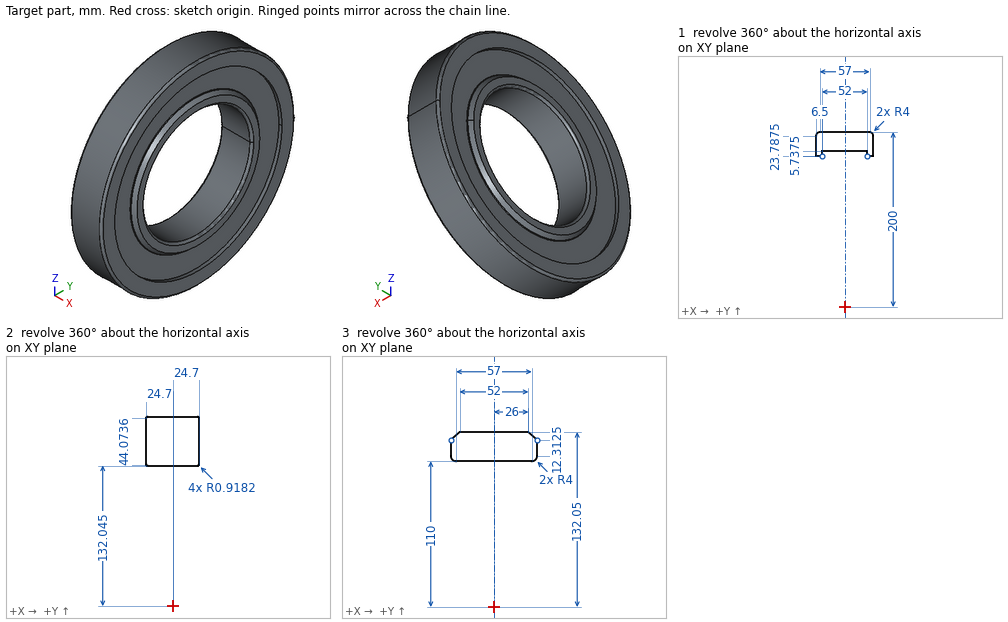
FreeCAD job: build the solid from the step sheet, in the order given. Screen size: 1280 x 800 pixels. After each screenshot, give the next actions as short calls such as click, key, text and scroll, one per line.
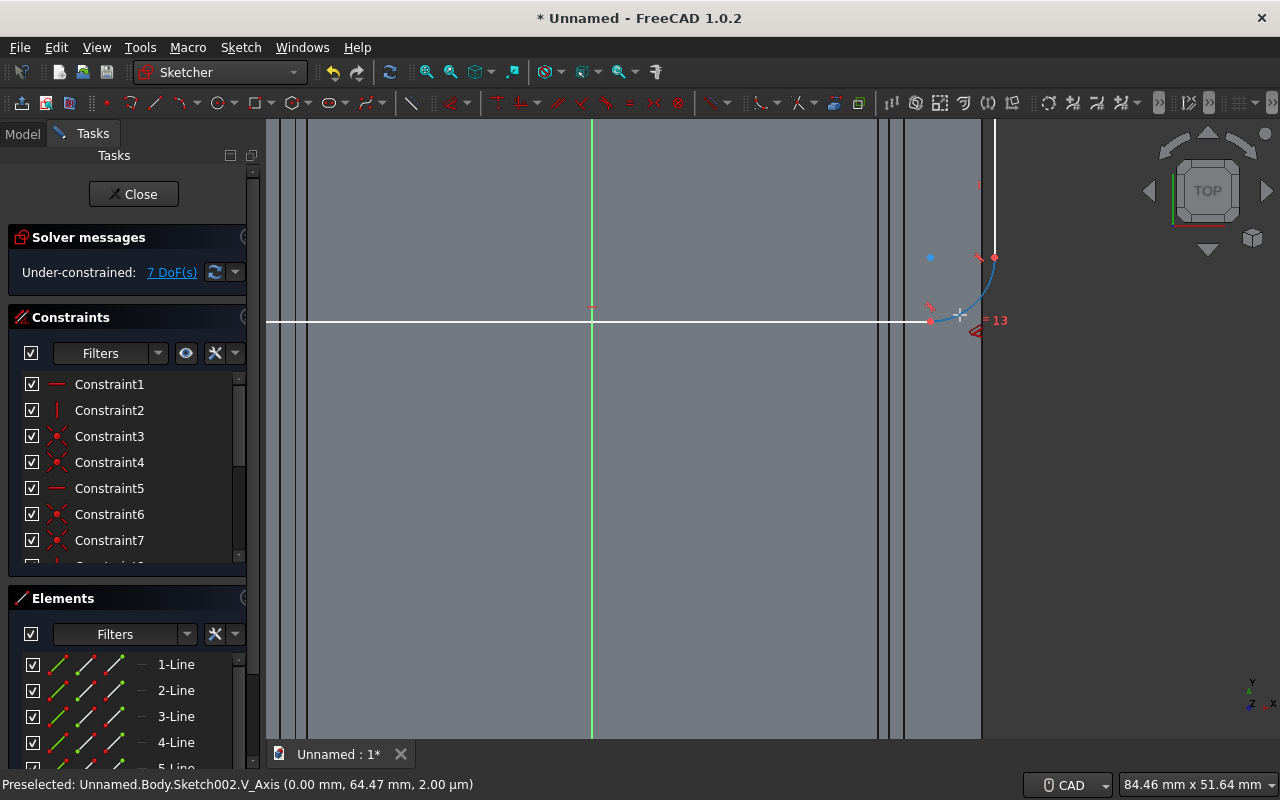
click(960, 315)
click(975, 343)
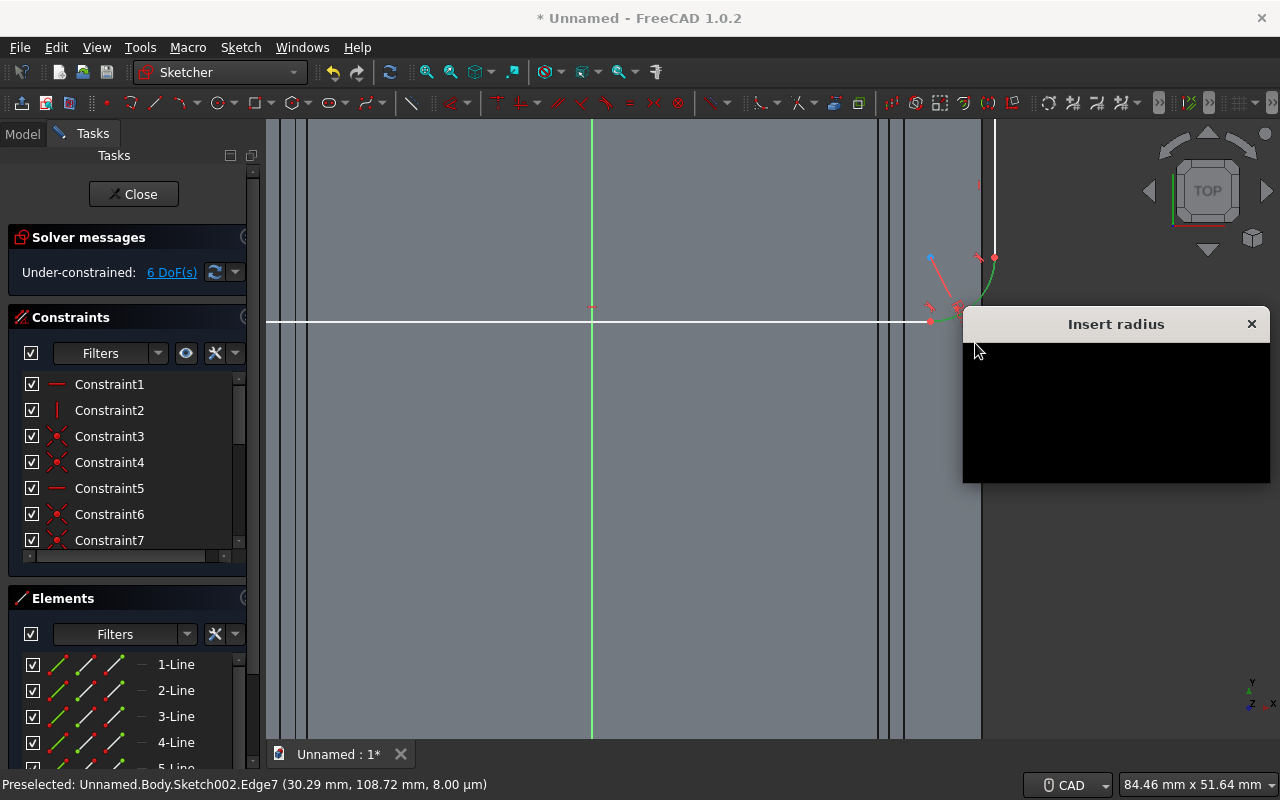
text(4)
key(Return)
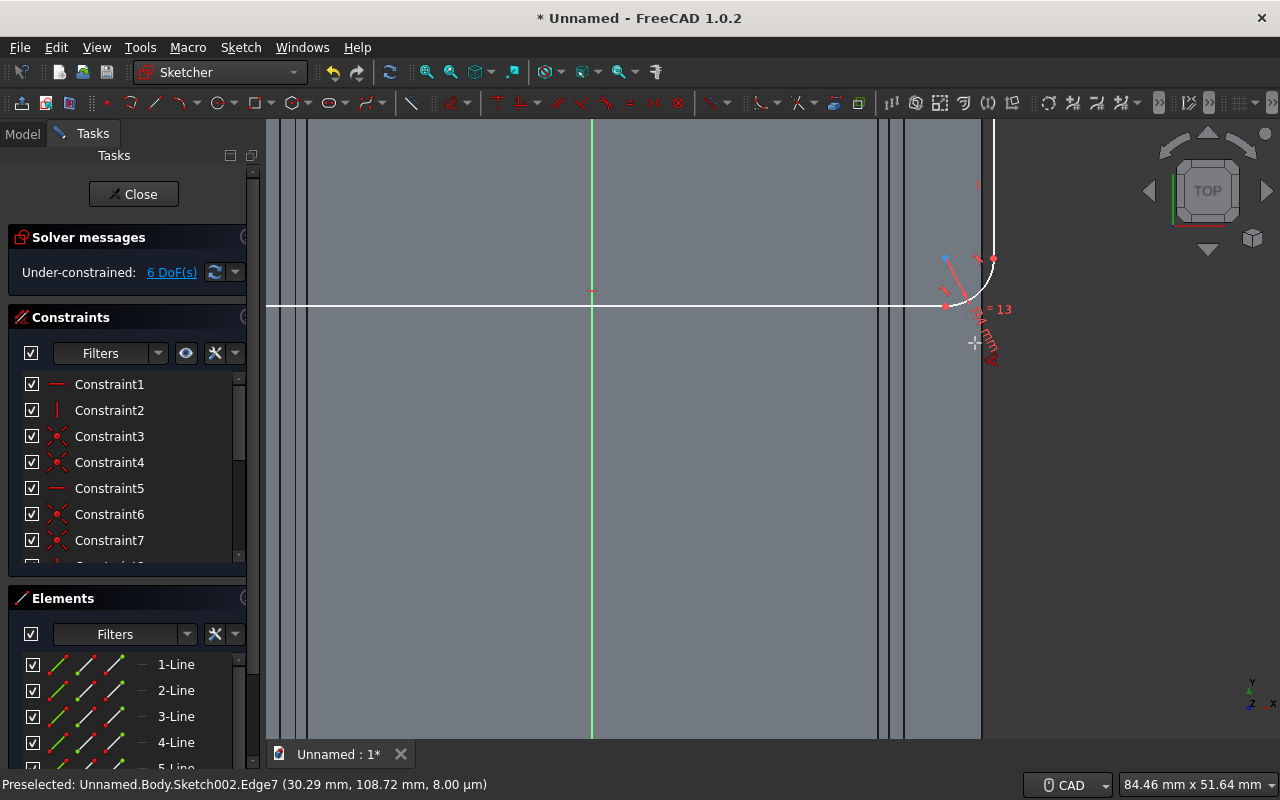
scroll(741, 298, down, 7)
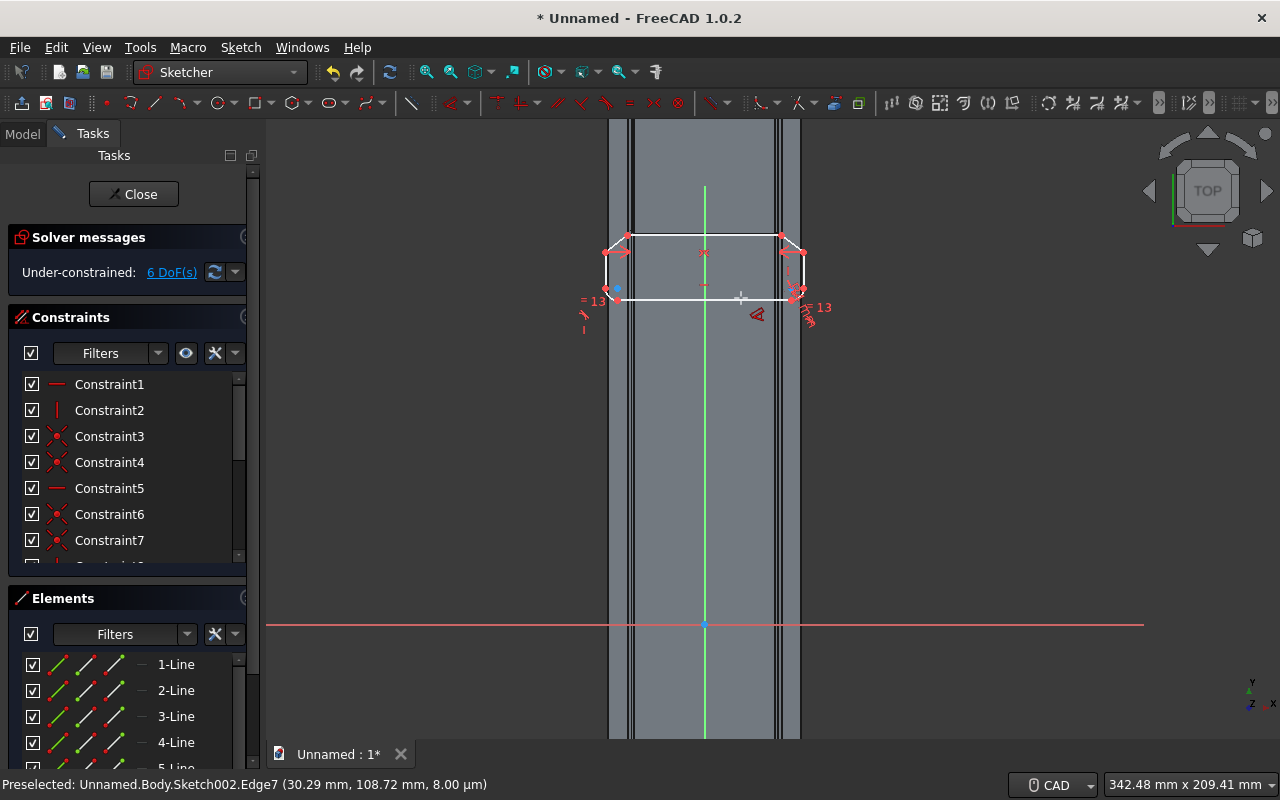
click(670, 300)
click(665, 266)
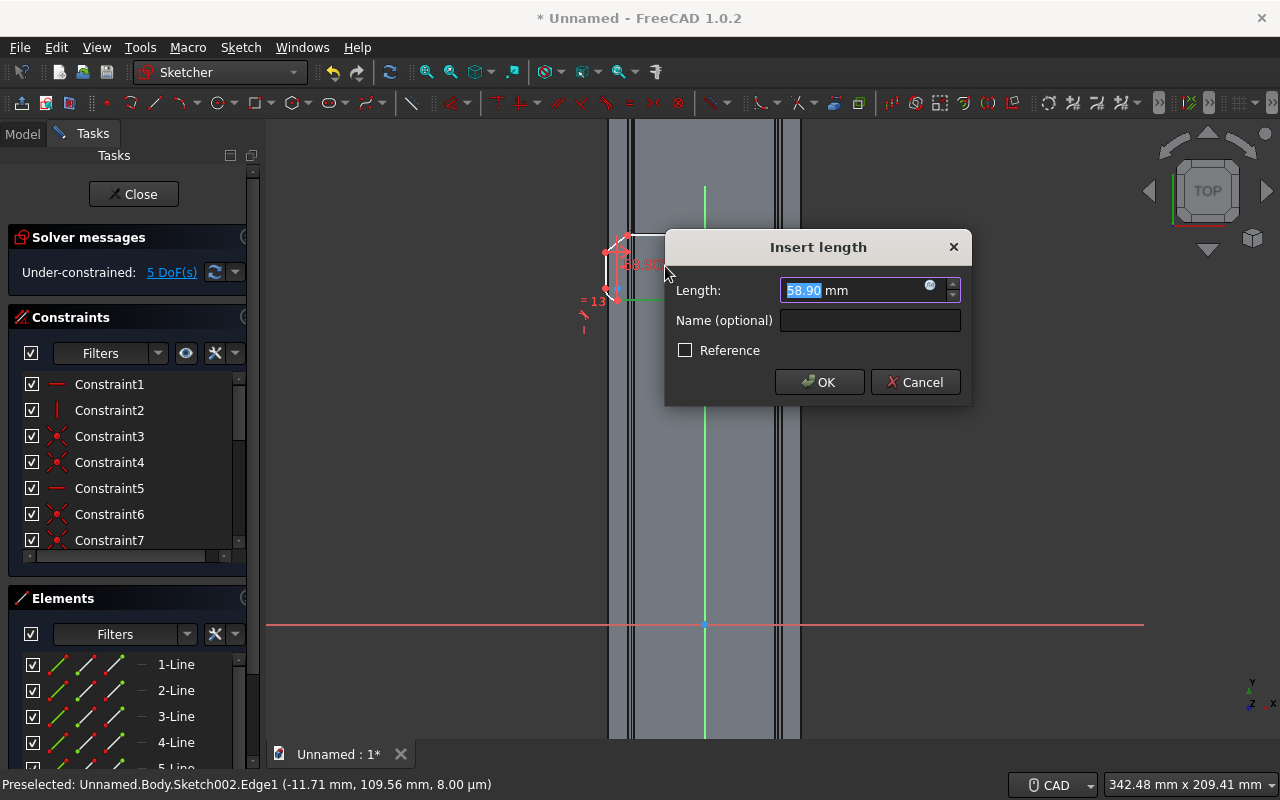
text(57)
key(Return)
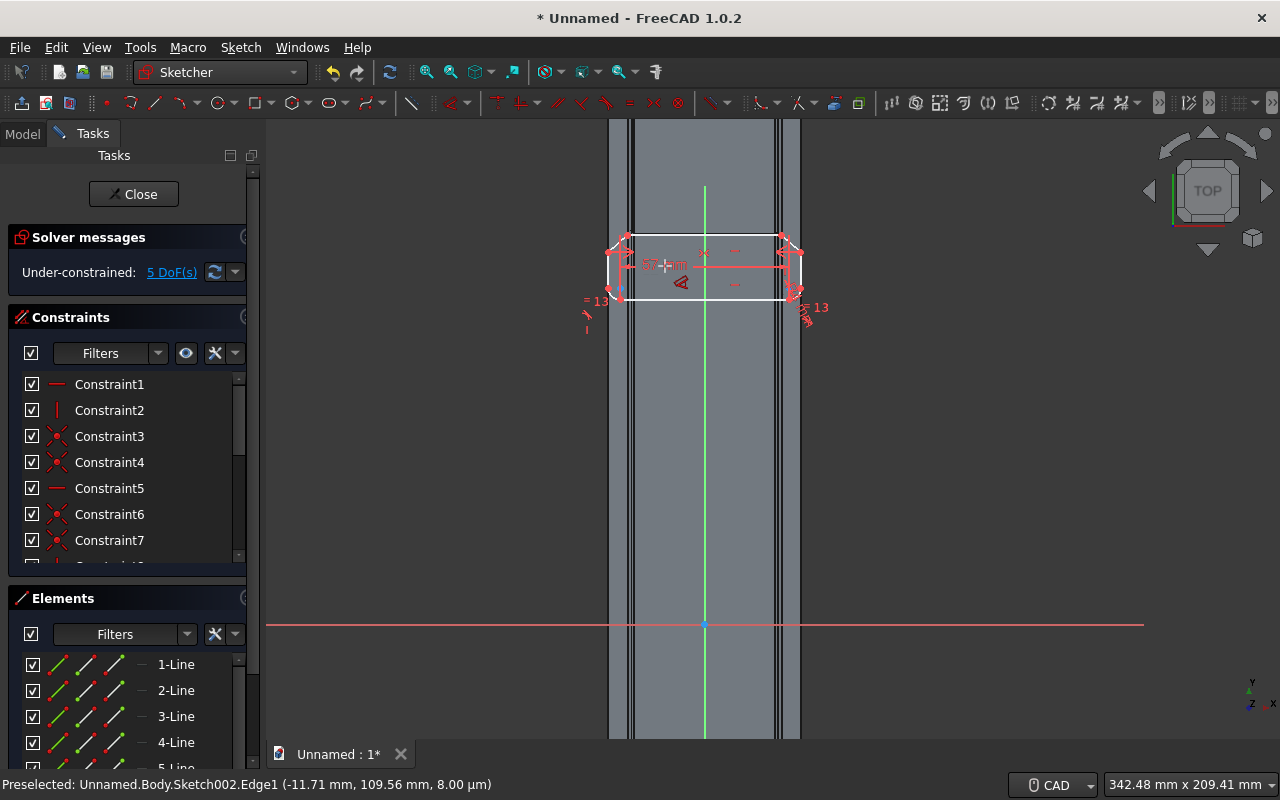
click(735, 235)
click(669, 201)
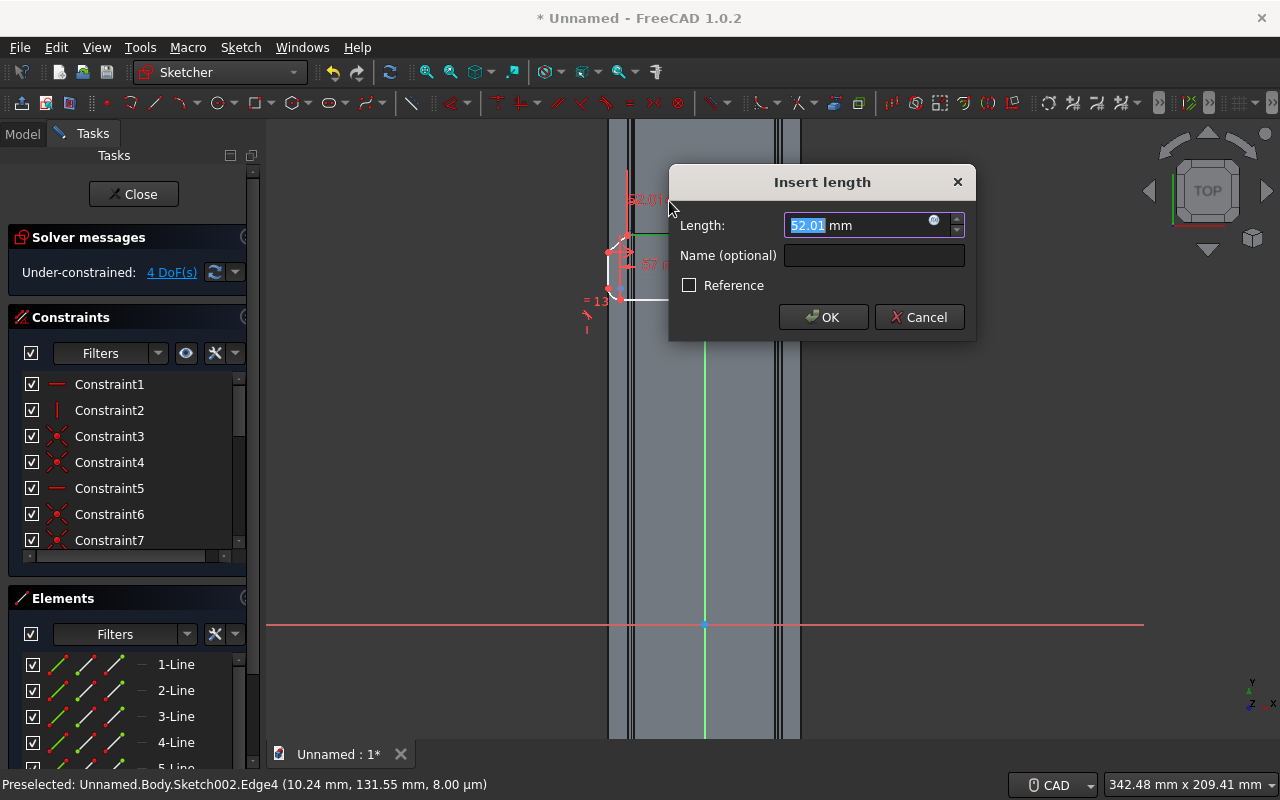
text(52)
key(Return)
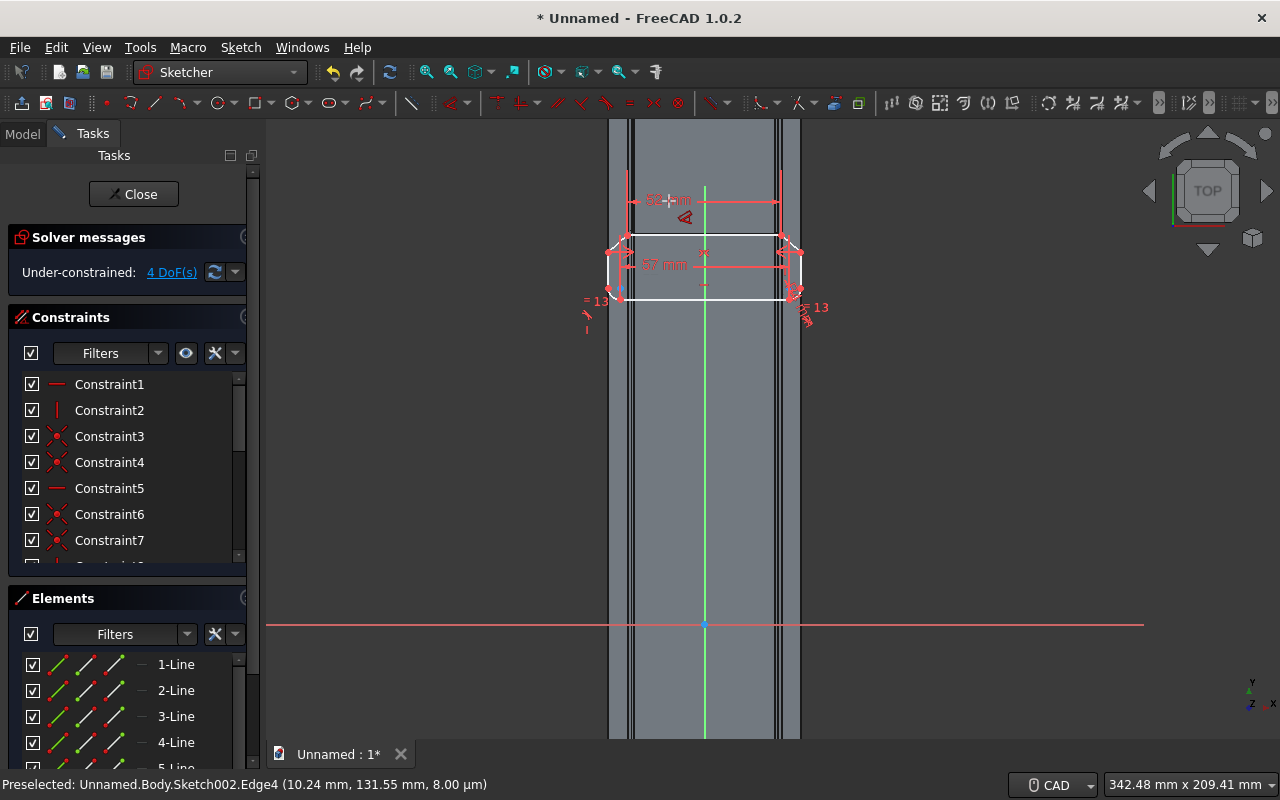
click(781, 235)
click(743, 659)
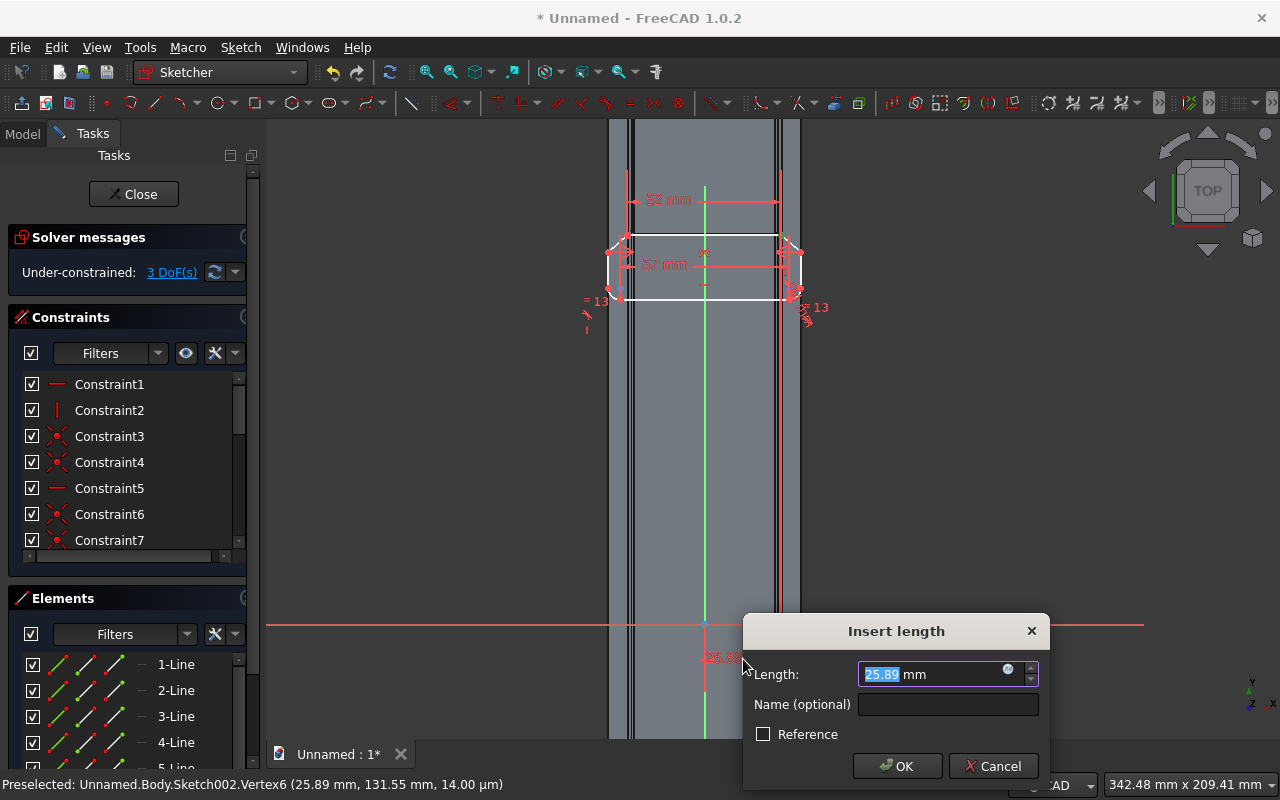
text(26)
key(Return)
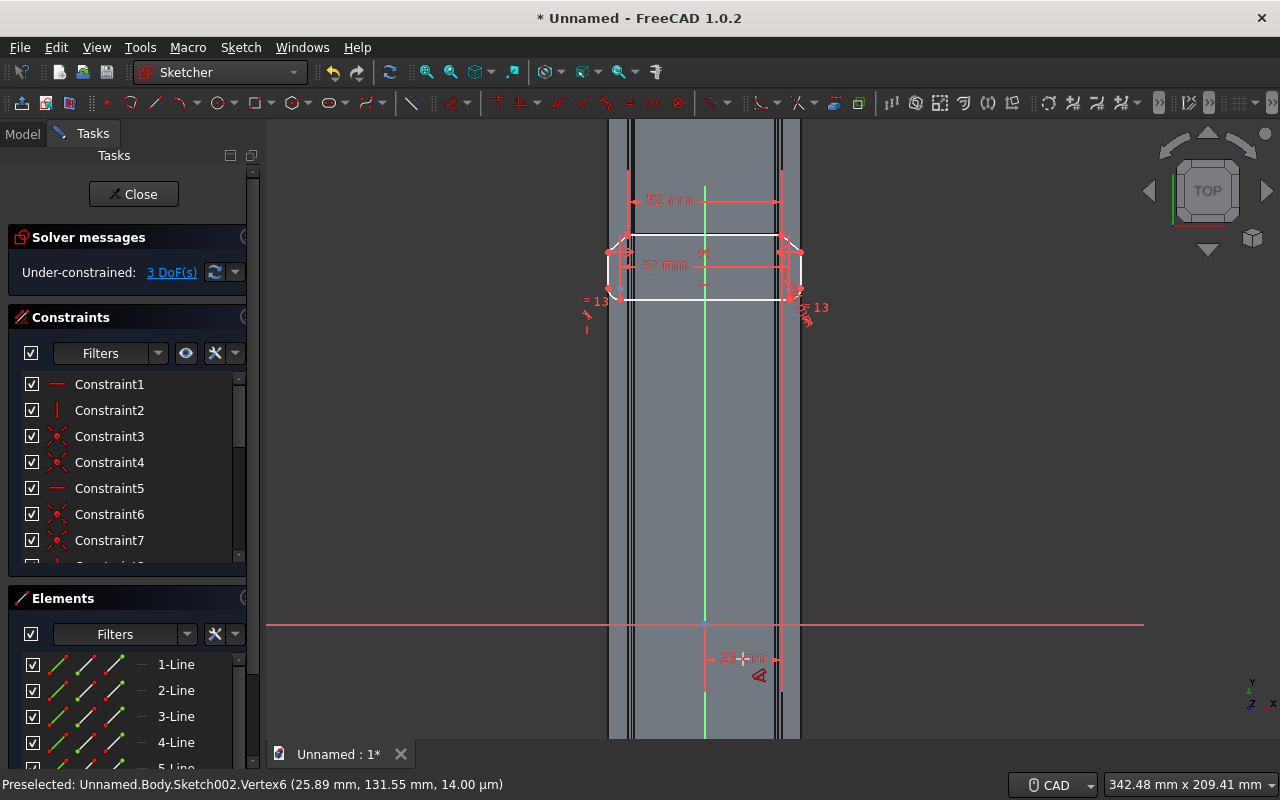
click(620, 300)
click(586, 462)